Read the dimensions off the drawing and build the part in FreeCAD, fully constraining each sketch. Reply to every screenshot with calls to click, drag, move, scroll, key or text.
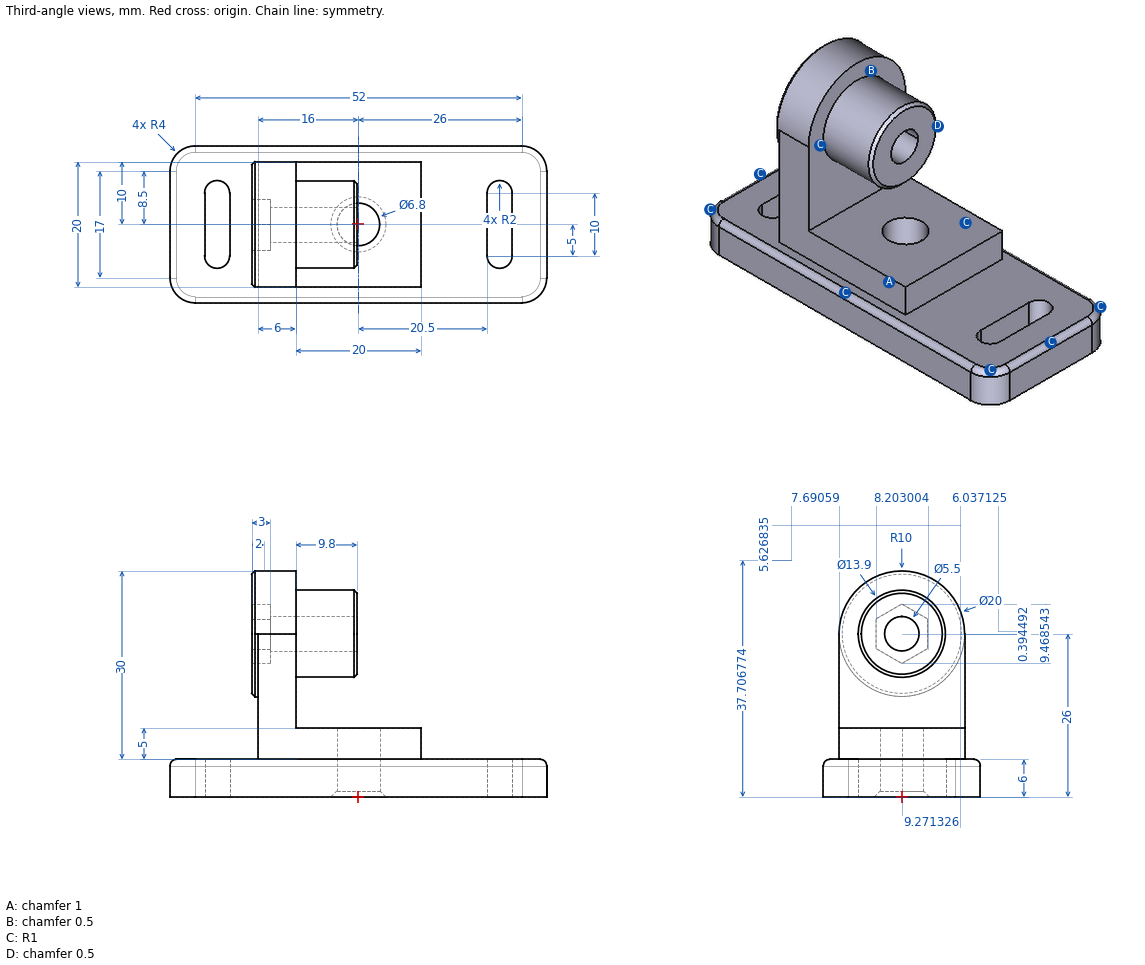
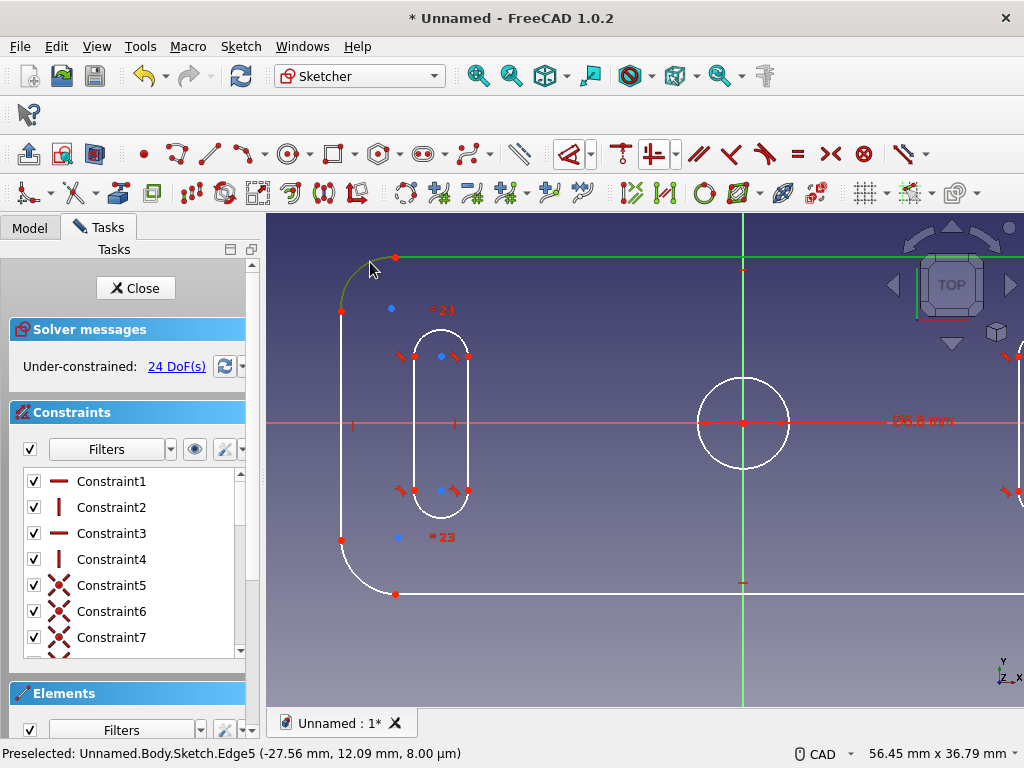
click(765, 154)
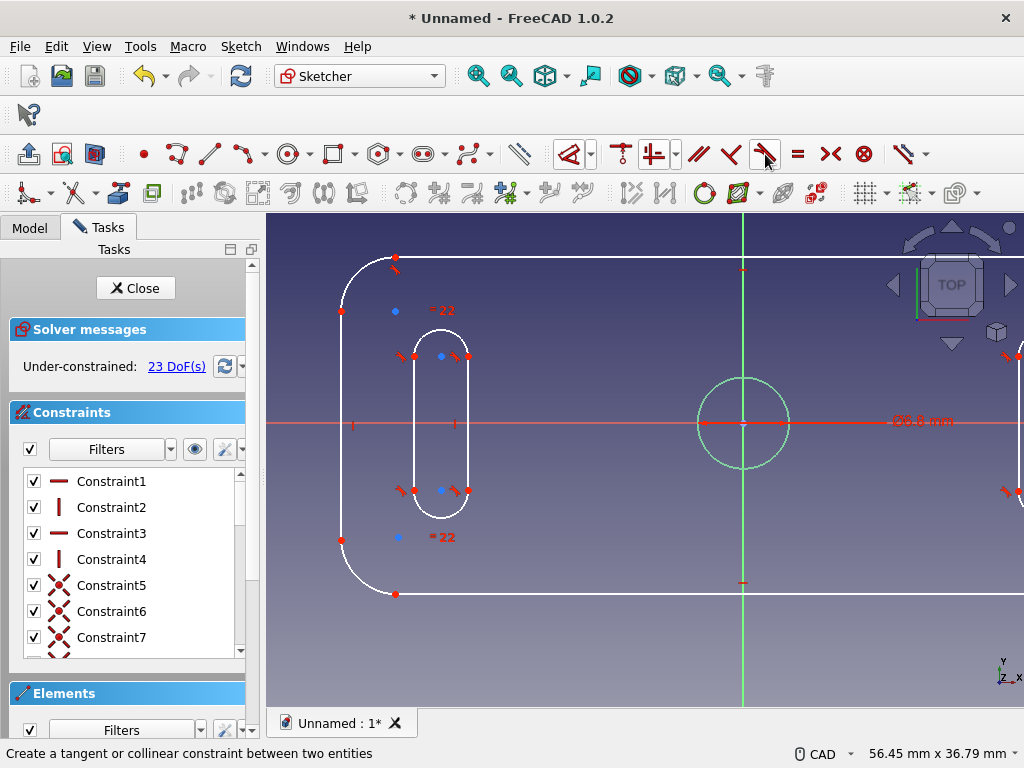
click(604, 257)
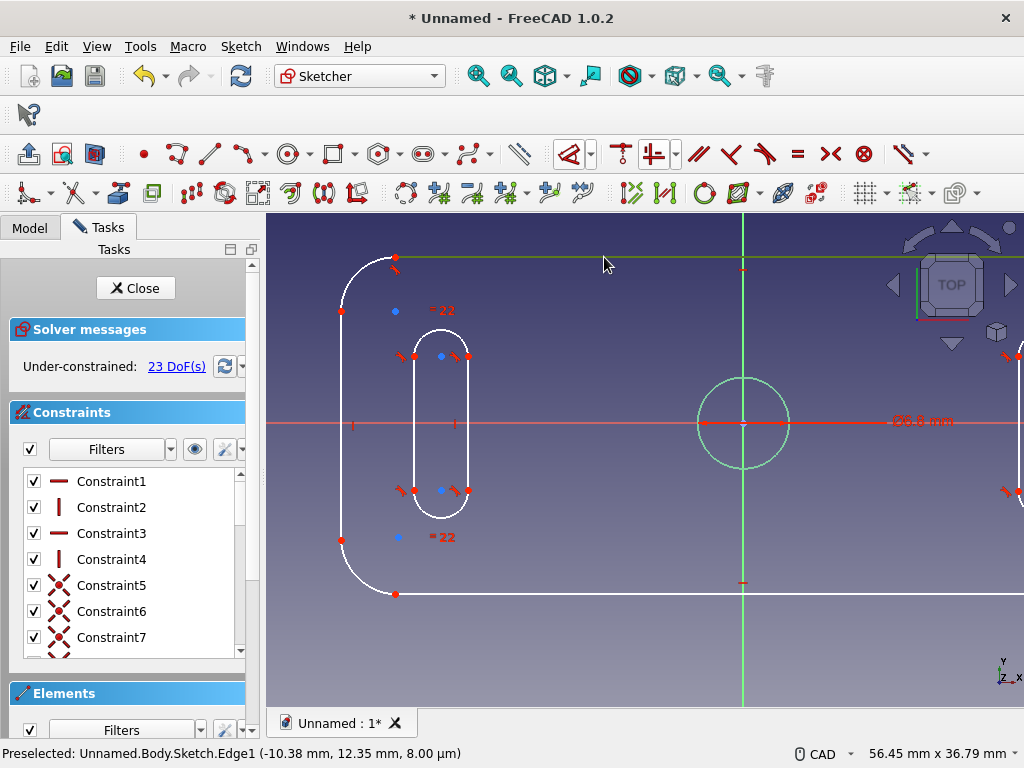
scroll(440, 490, down, 4)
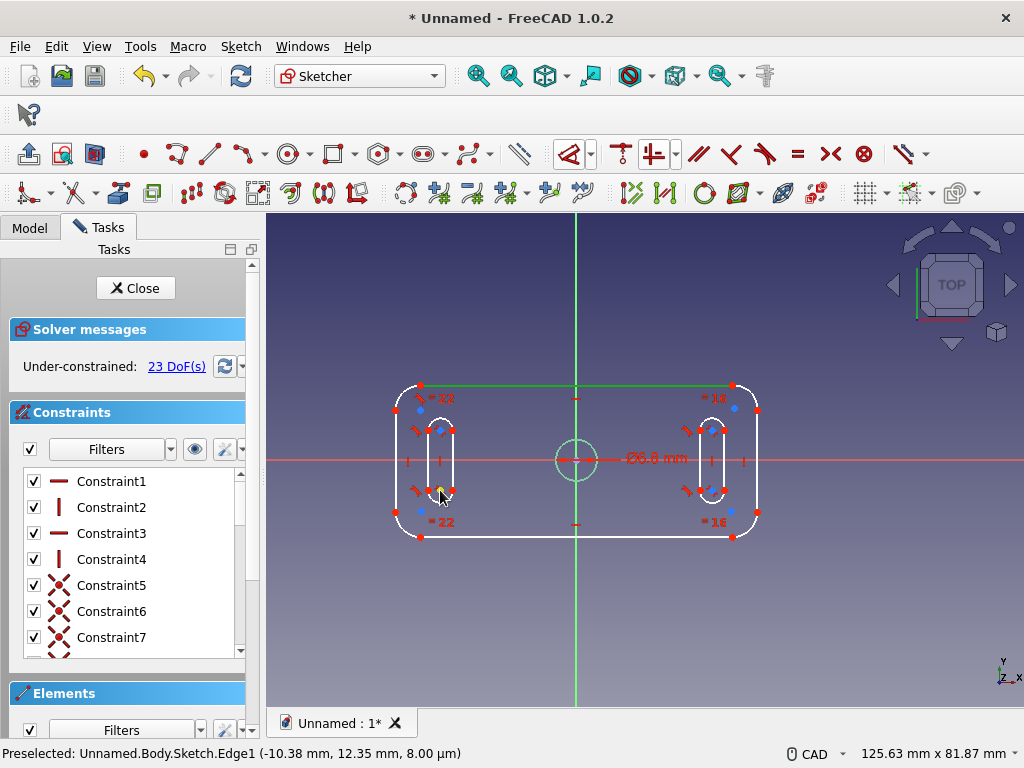
click(755, 399)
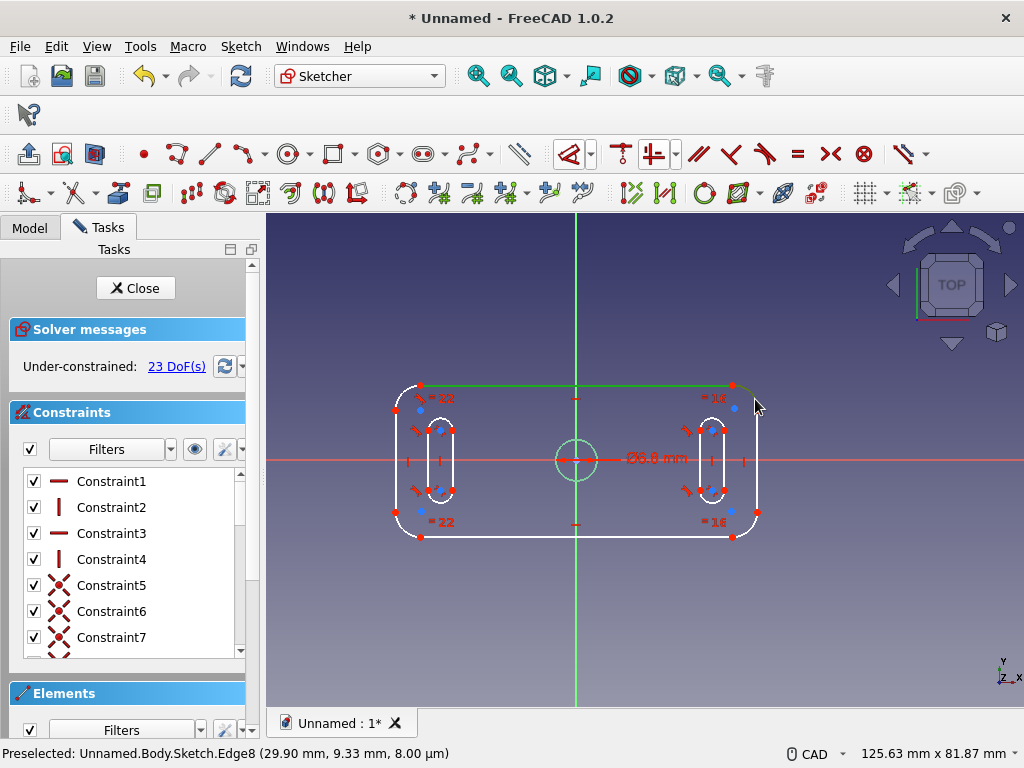
key(t)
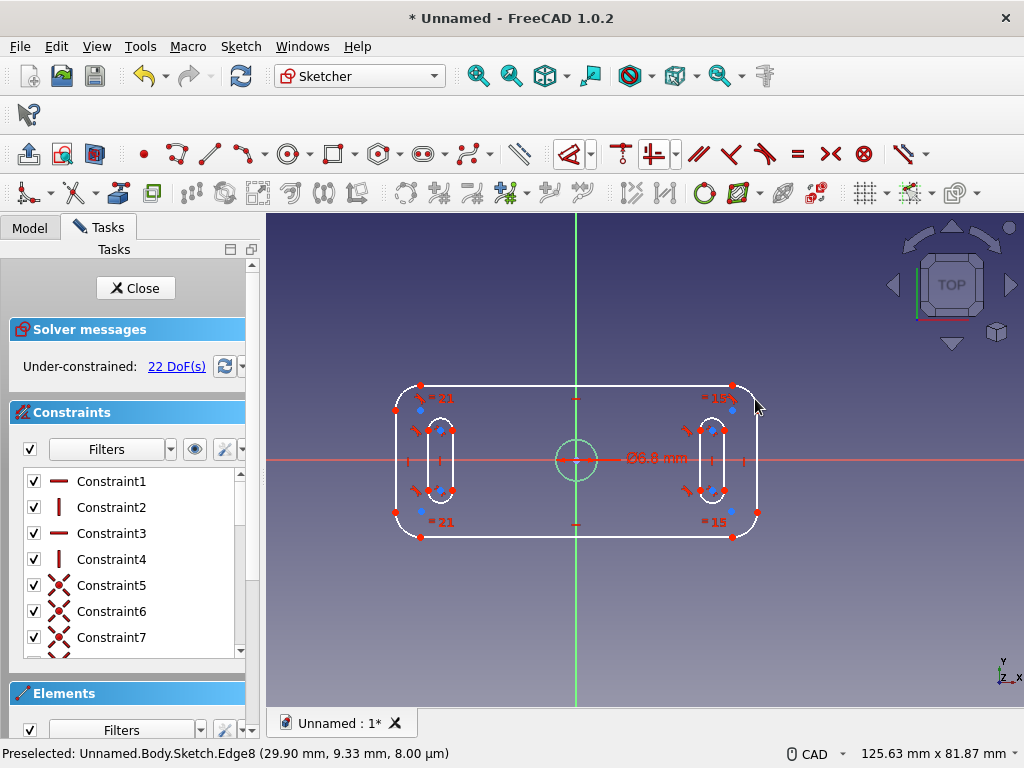
click(396, 441)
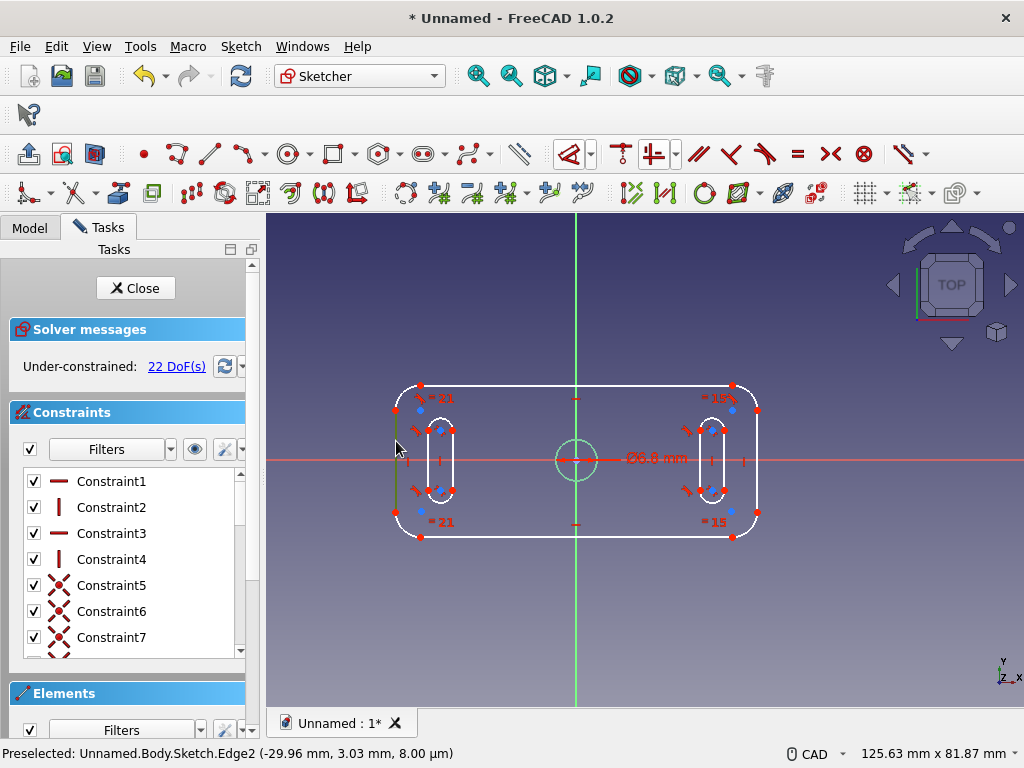
click(409, 388)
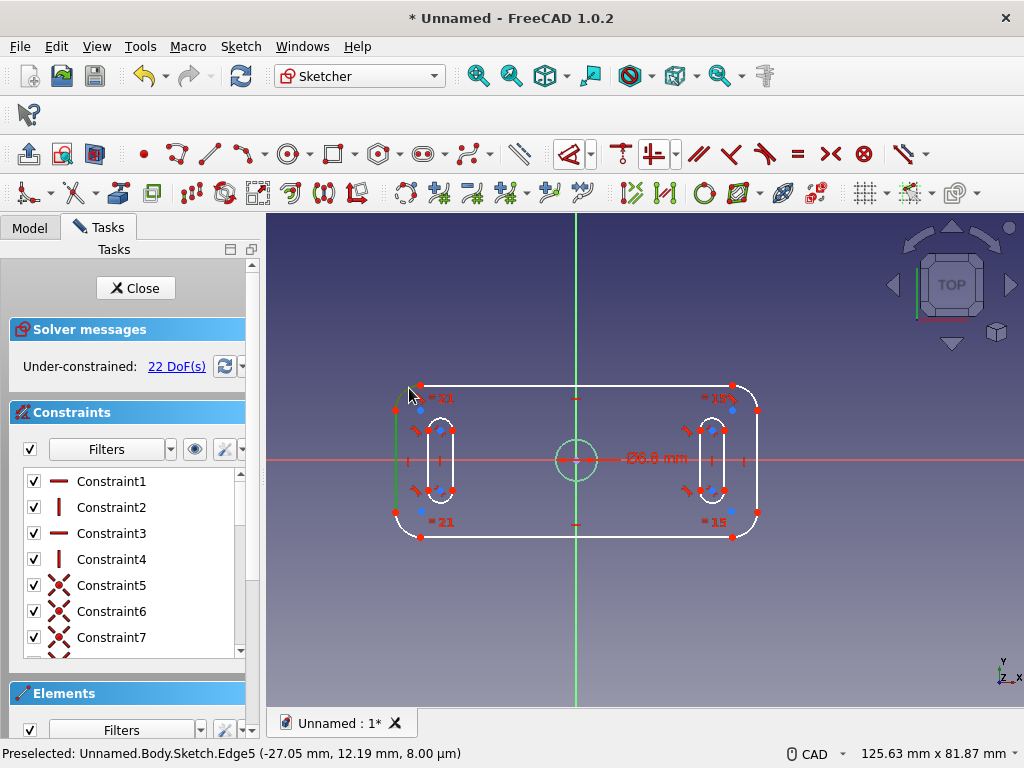
click(765, 154)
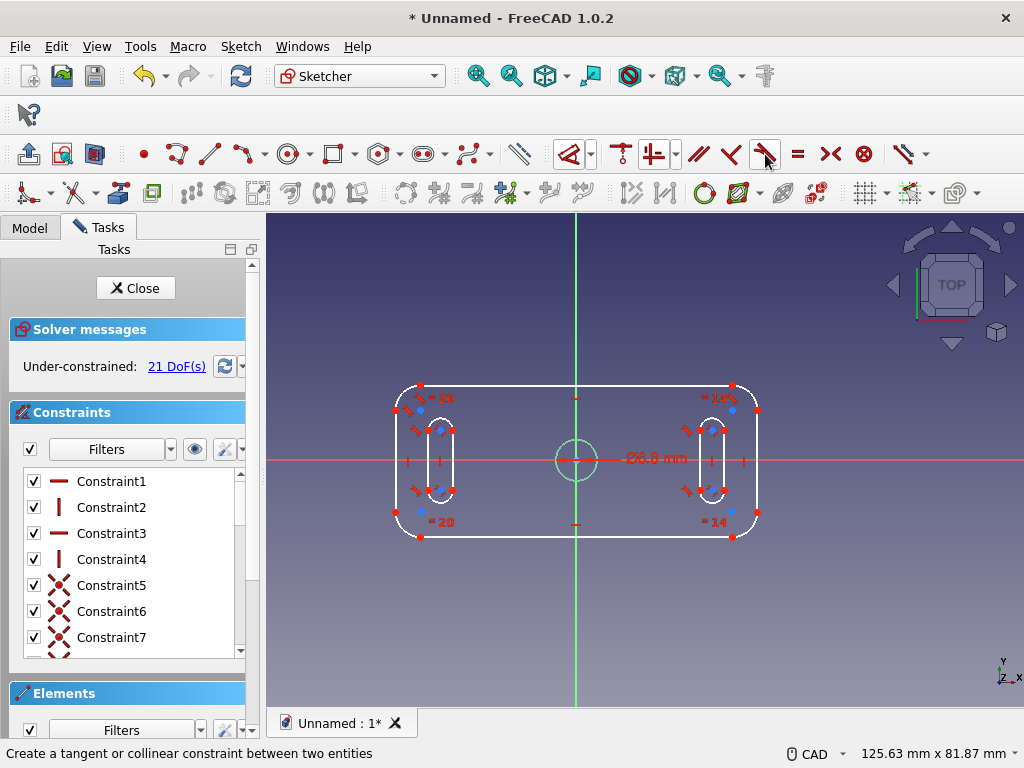
click(396, 441)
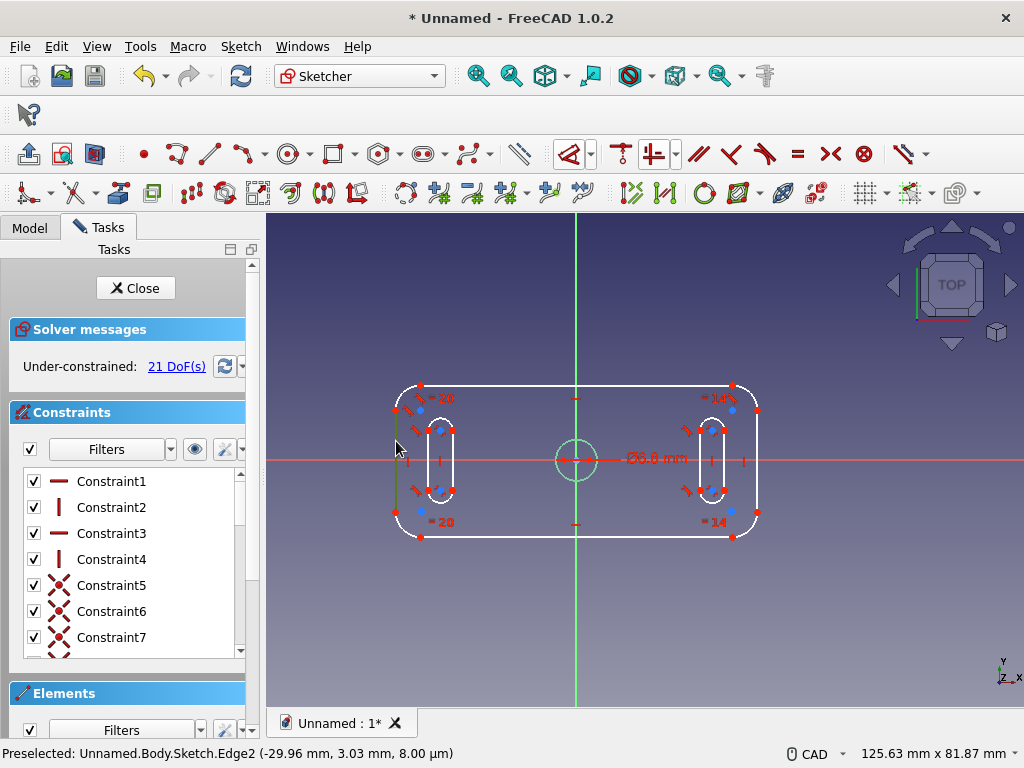
scroll(399, 524, up, 2)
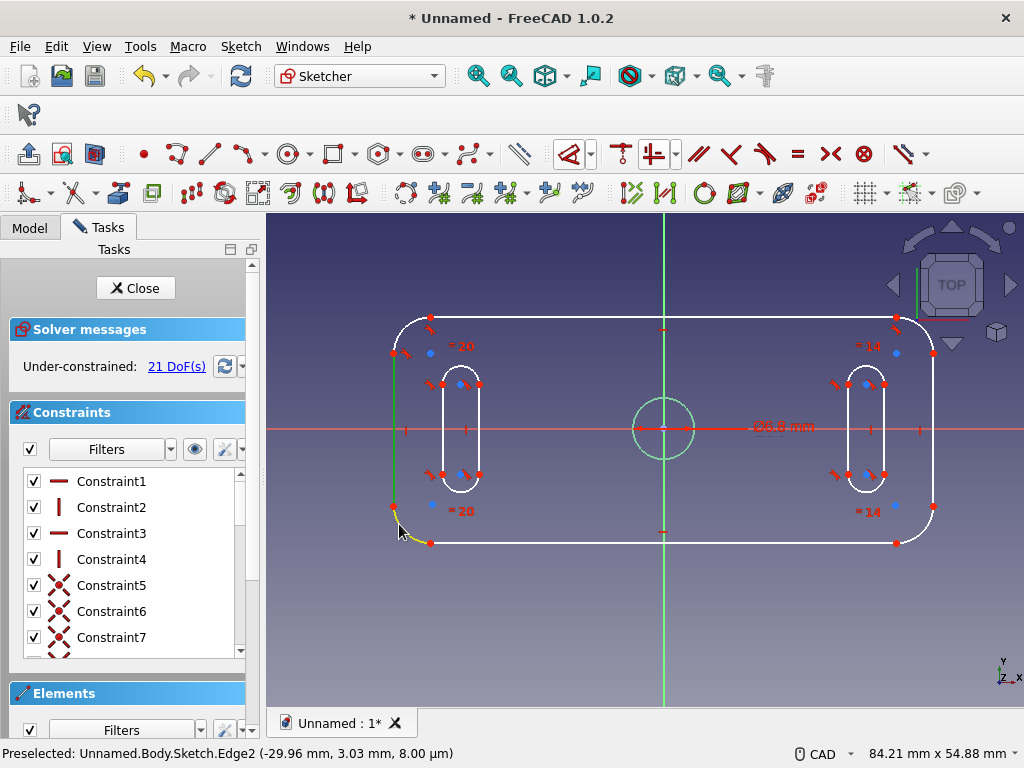
click(398, 523)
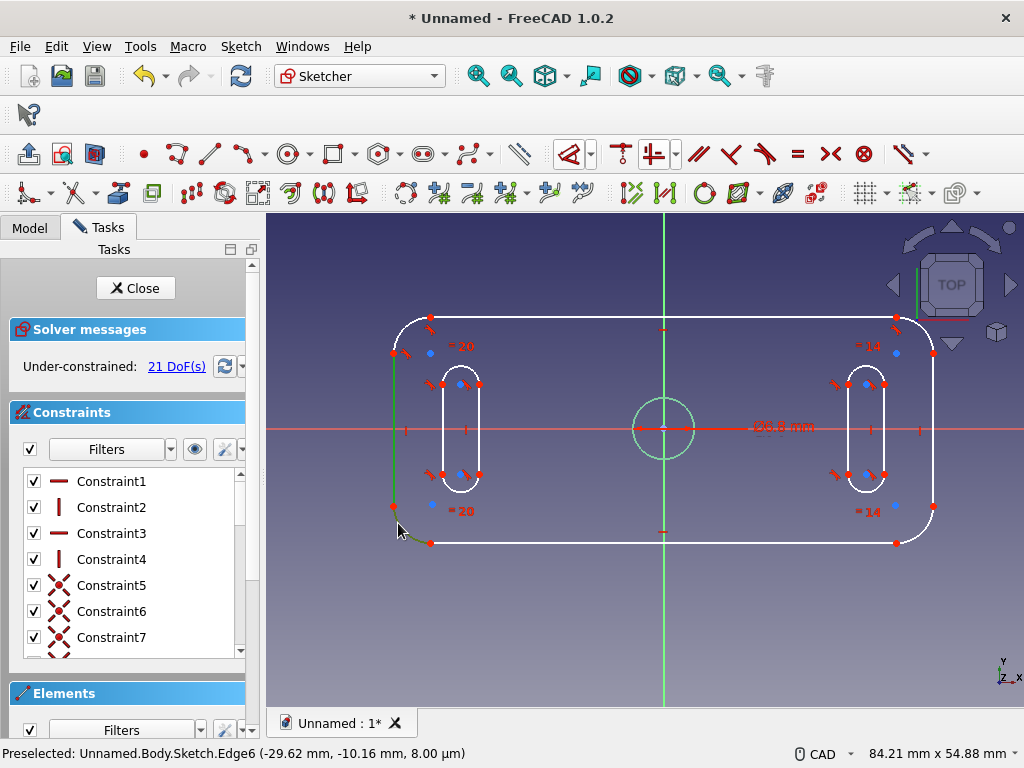
click(765, 154)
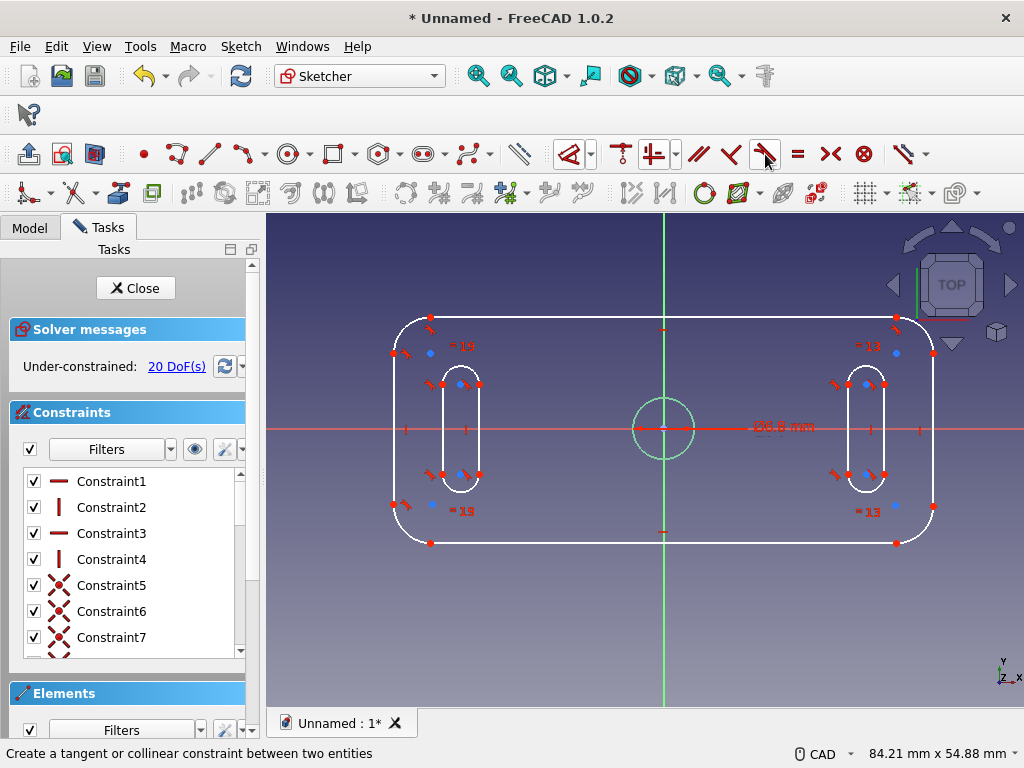
click(570, 543)